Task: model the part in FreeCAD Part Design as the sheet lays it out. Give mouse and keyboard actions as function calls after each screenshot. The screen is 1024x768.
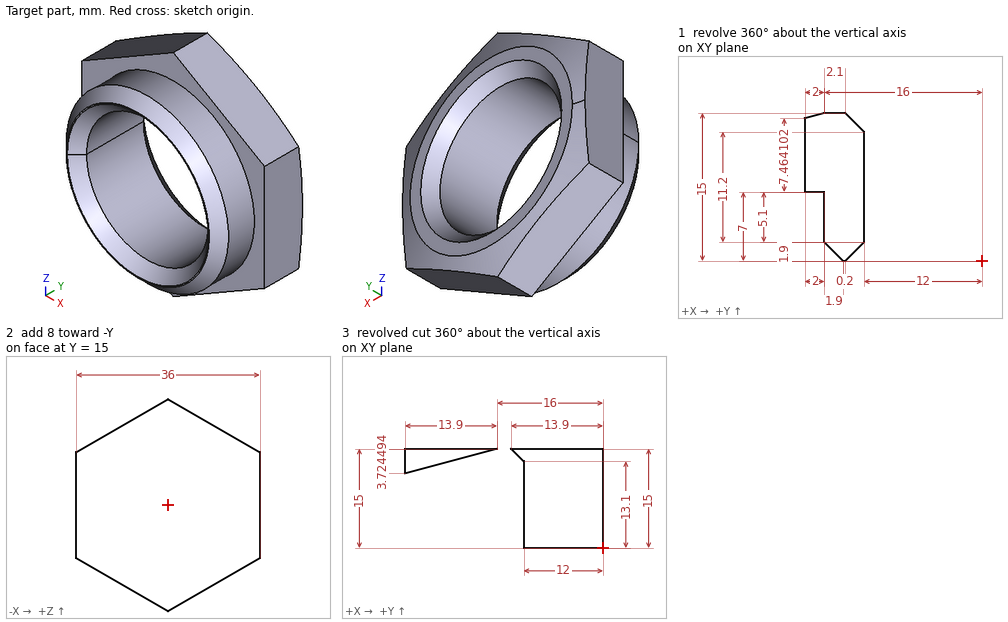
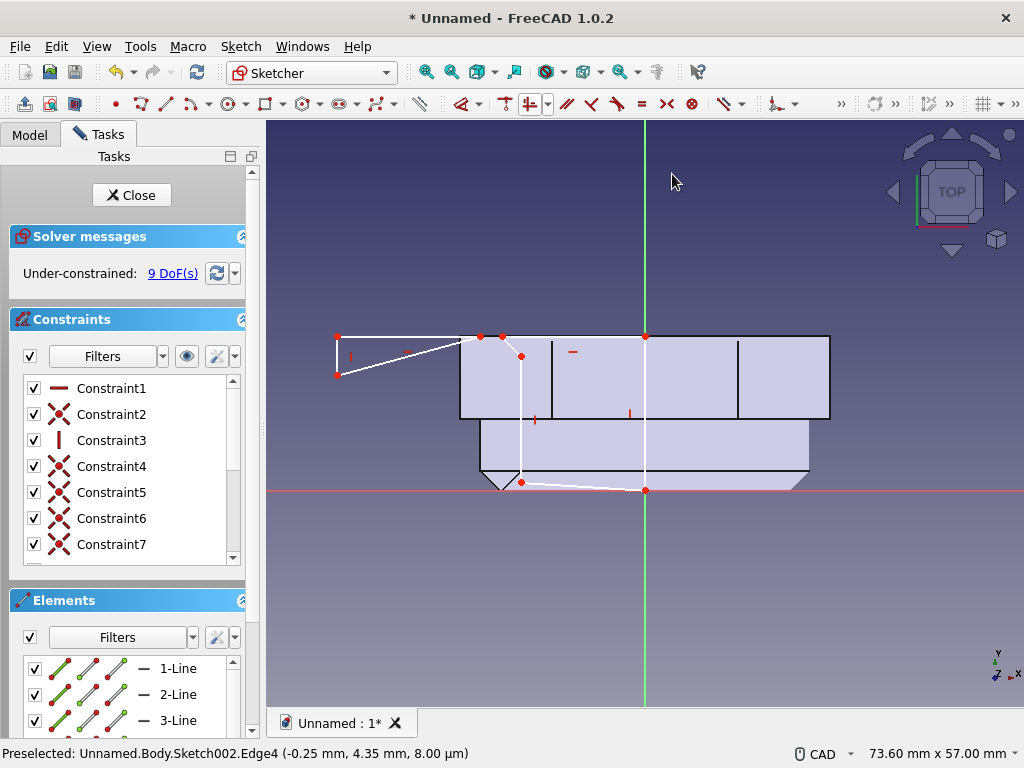
click(608, 488)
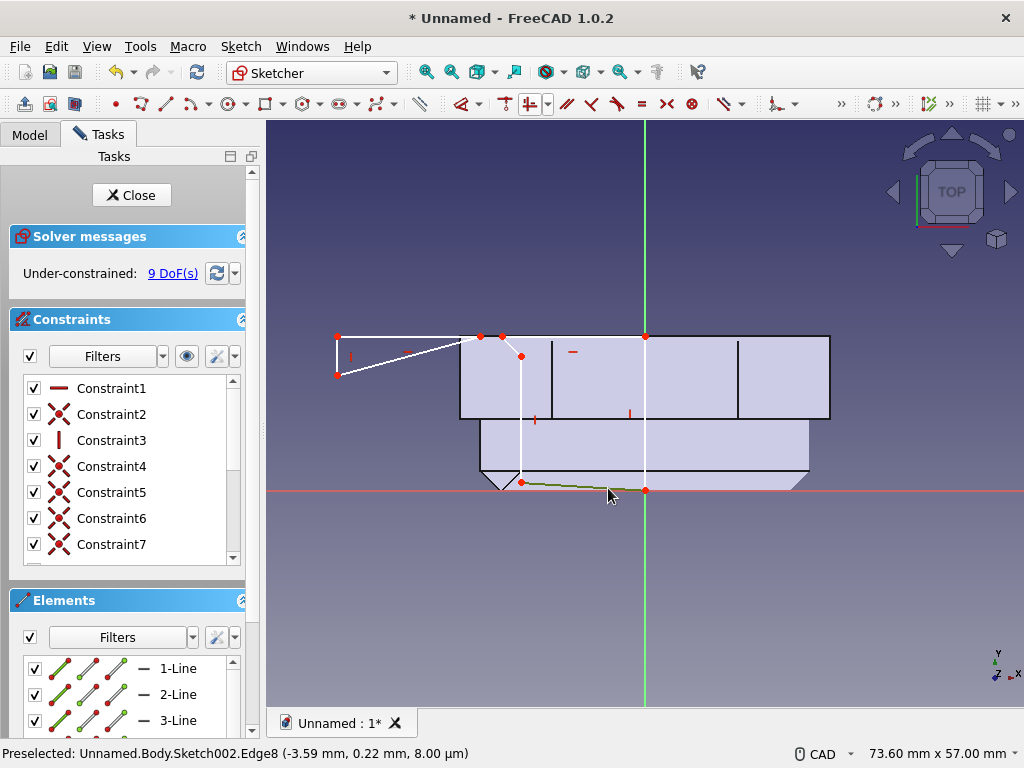
key(h)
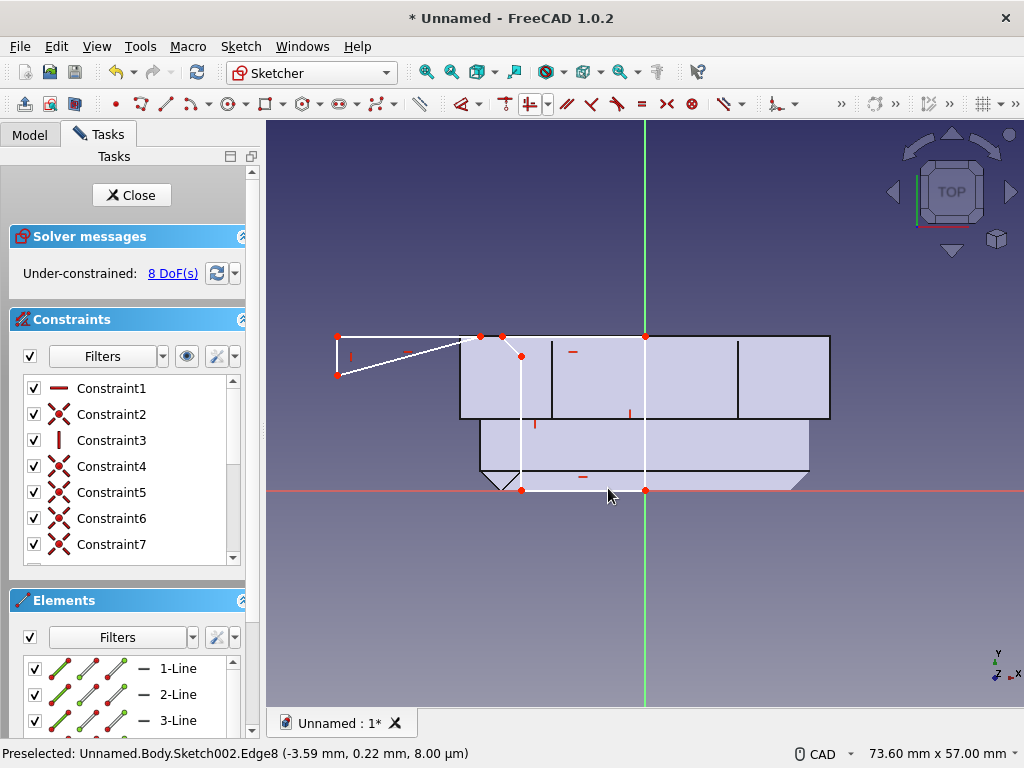
click(460, 104)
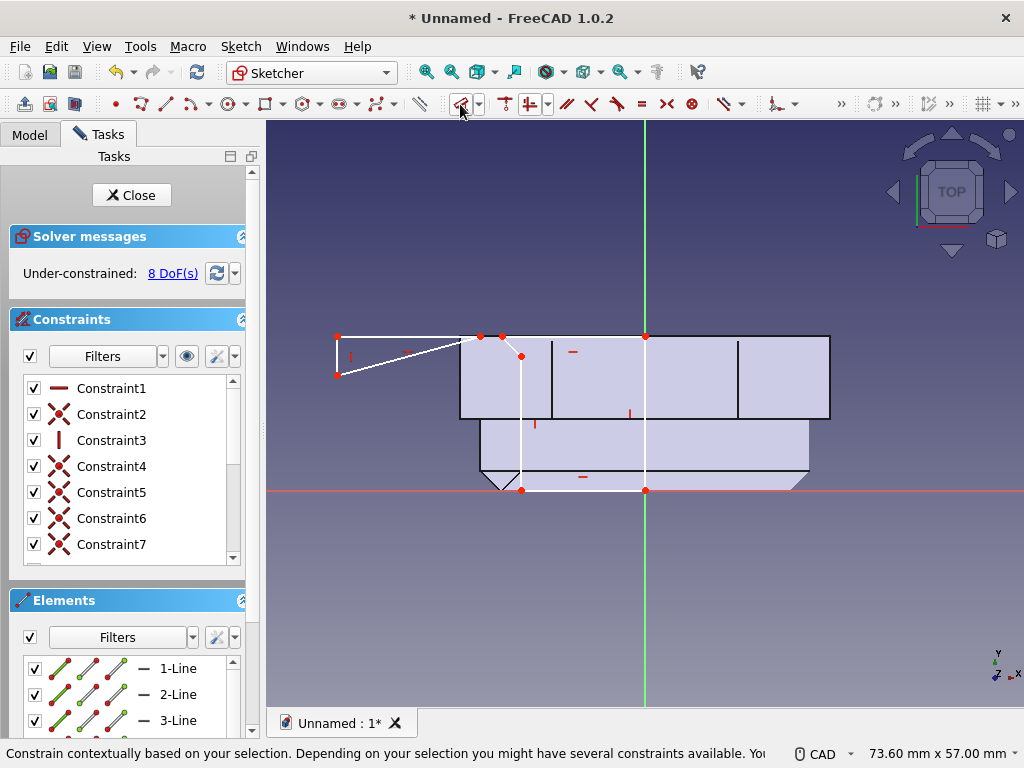
click(645, 445)
click(679, 414)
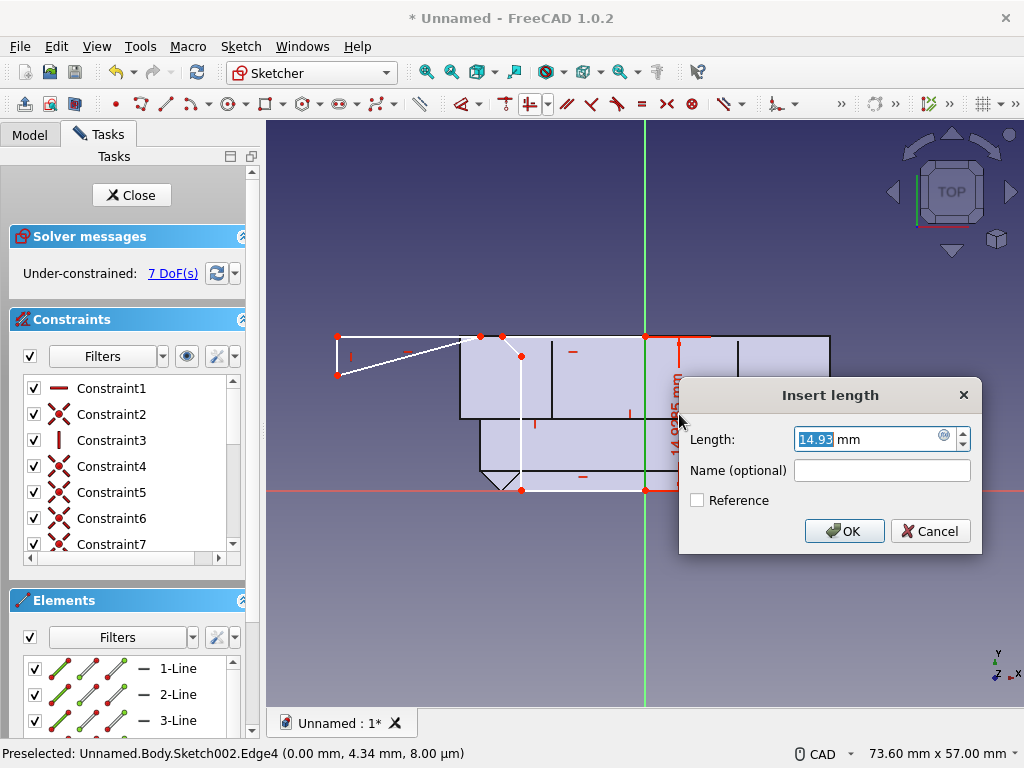
text(15)
key(Return)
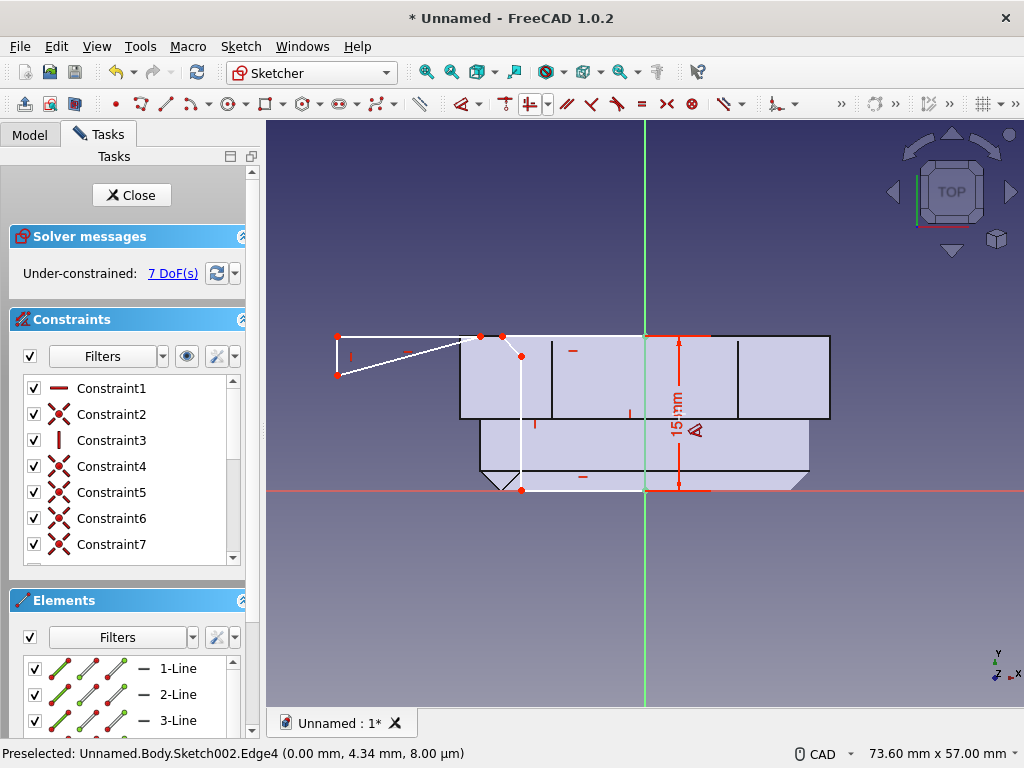
click(558, 491)
click(583, 525)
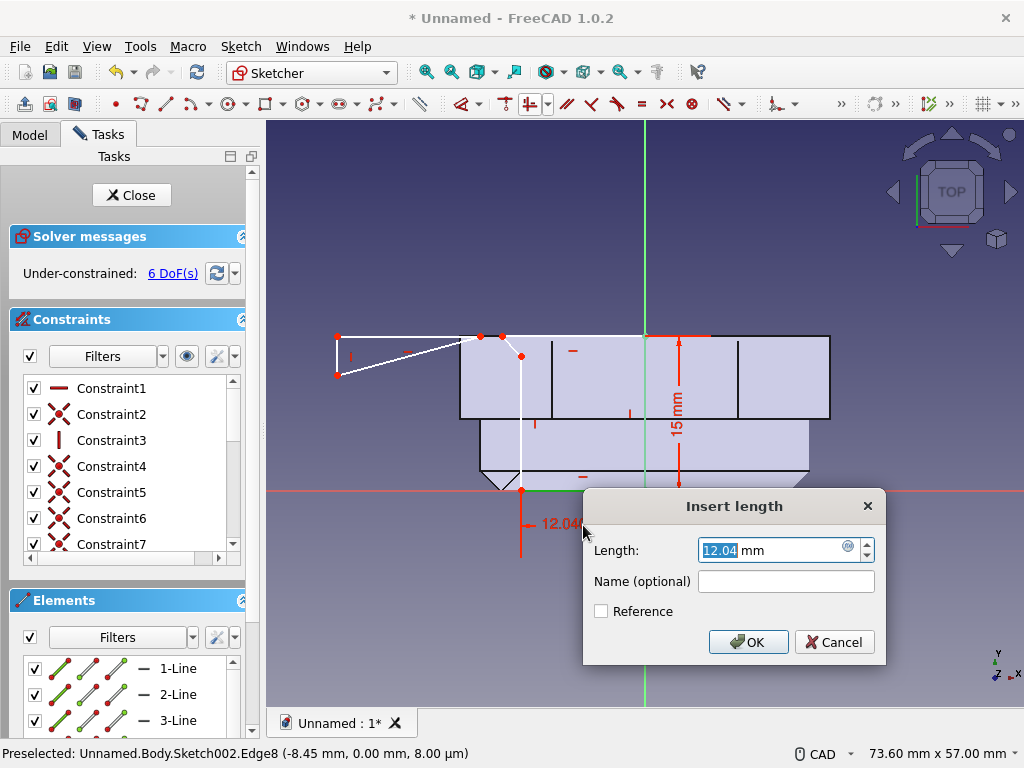
text(12)
key(Return)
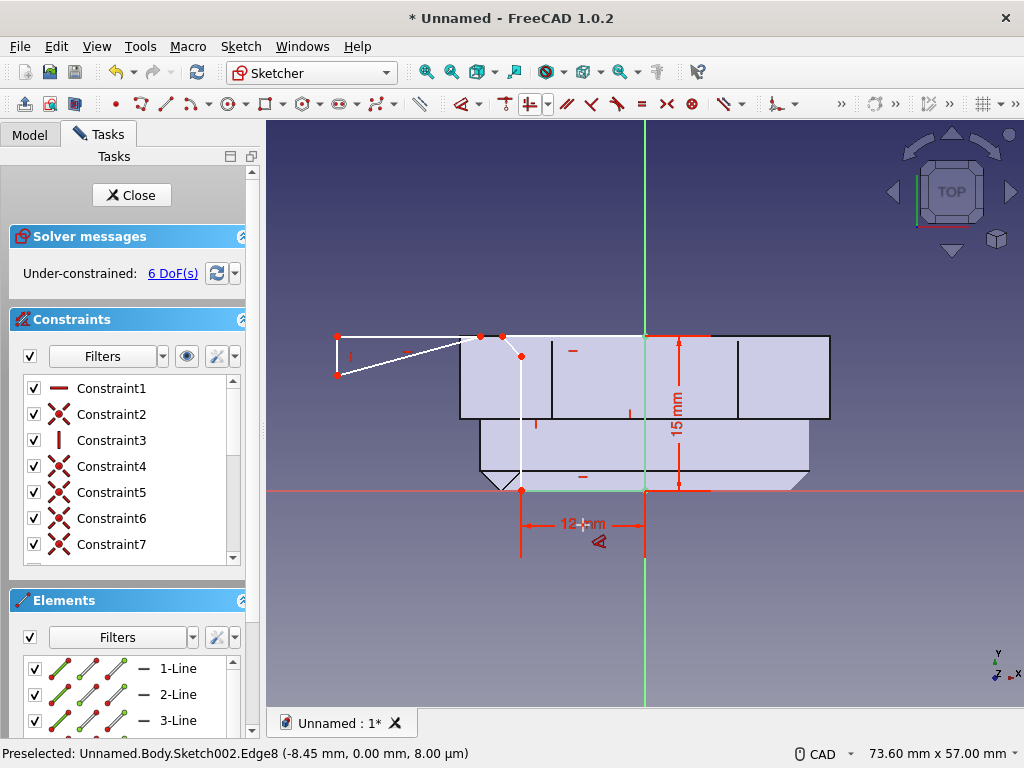
click(480, 337)
click(505, 525)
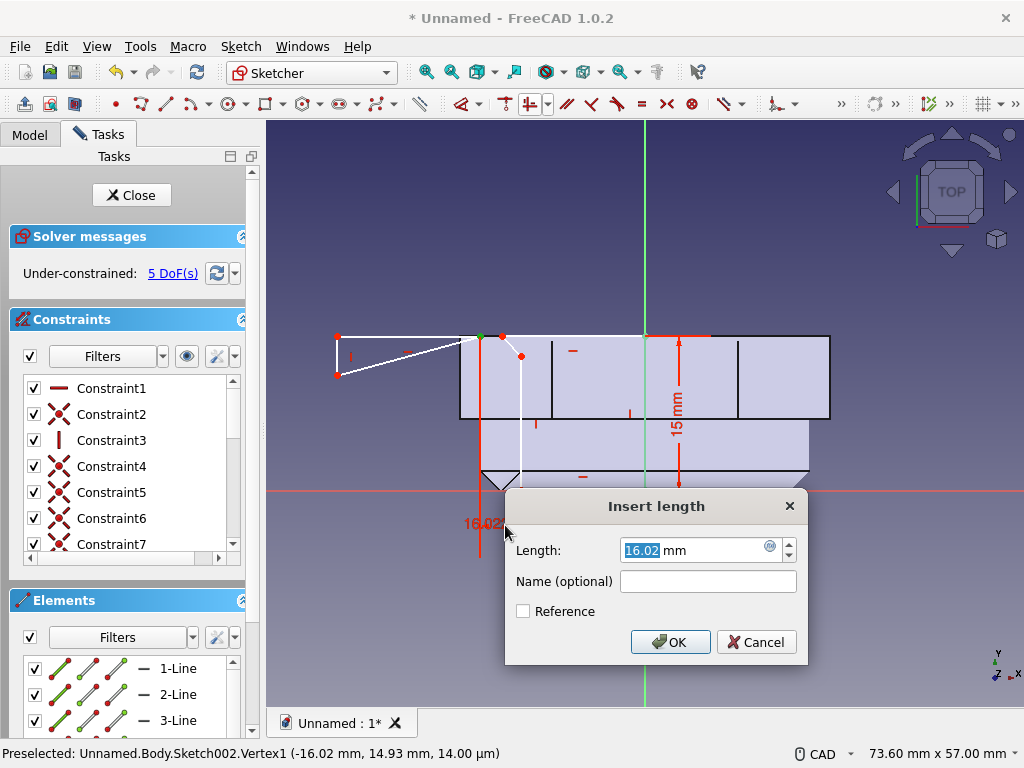
text(16)
key(Return)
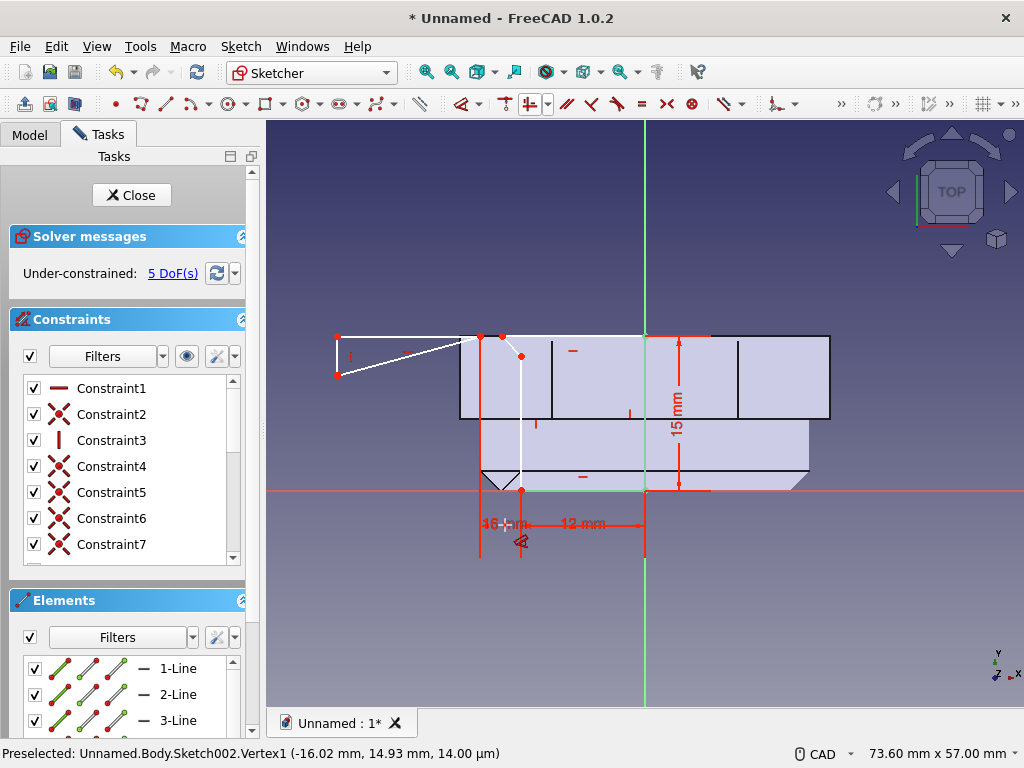
click(480, 337)
click(679, 379)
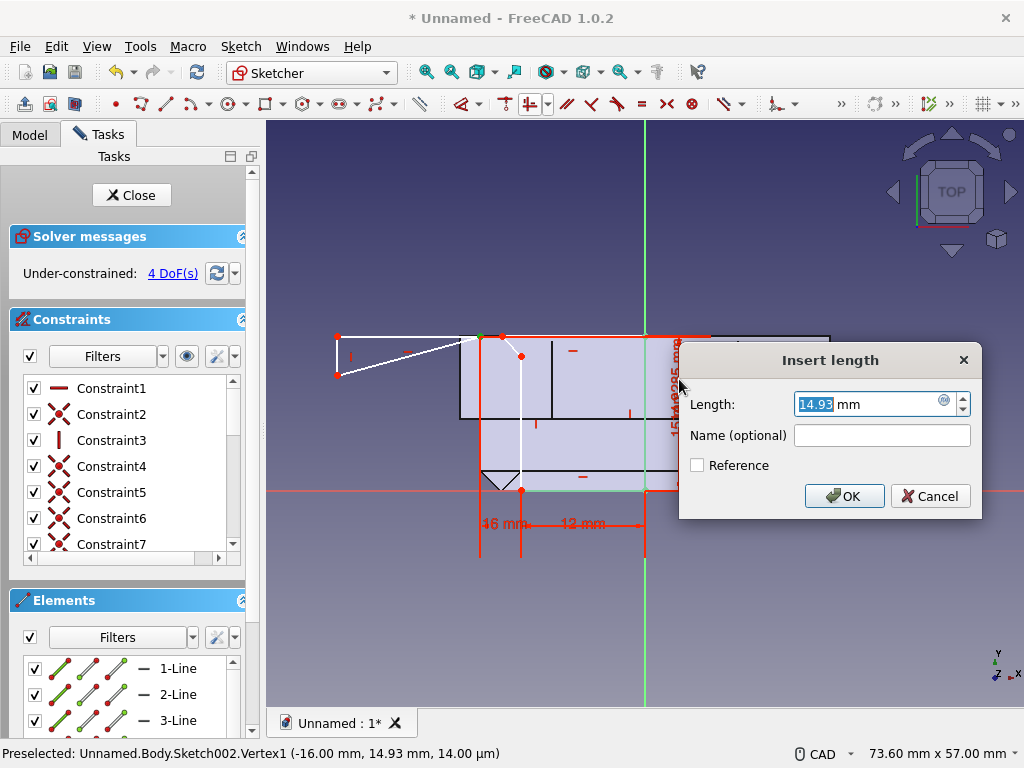
text(15)
key(Return)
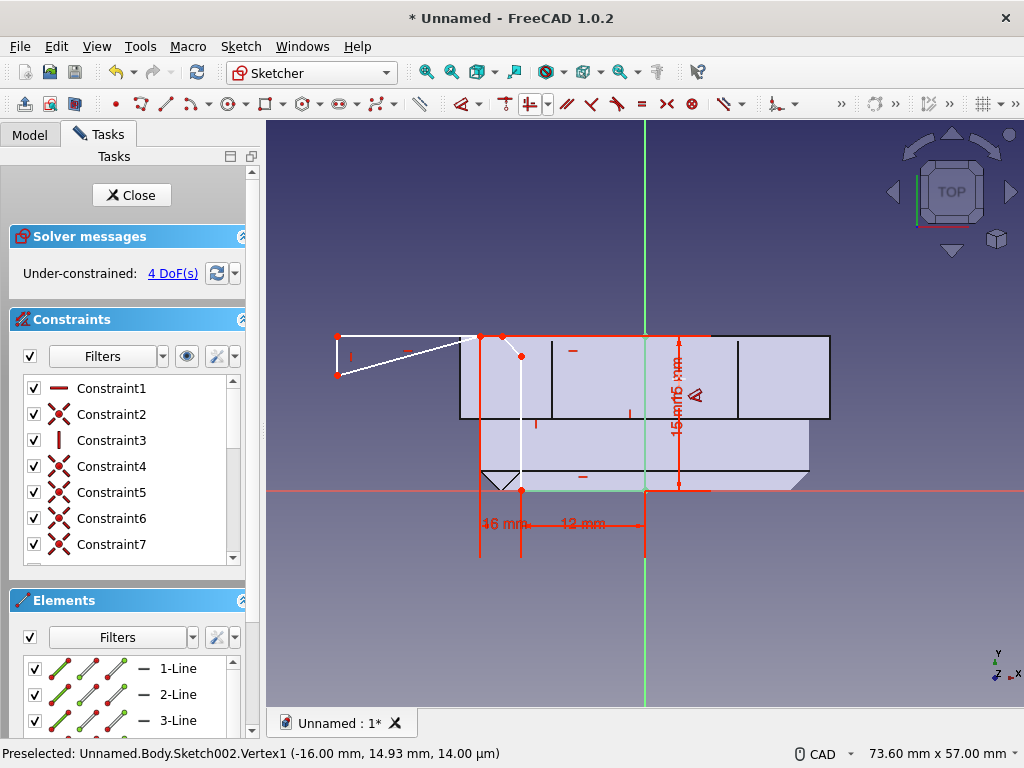
click(437, 336)
click(409, 302)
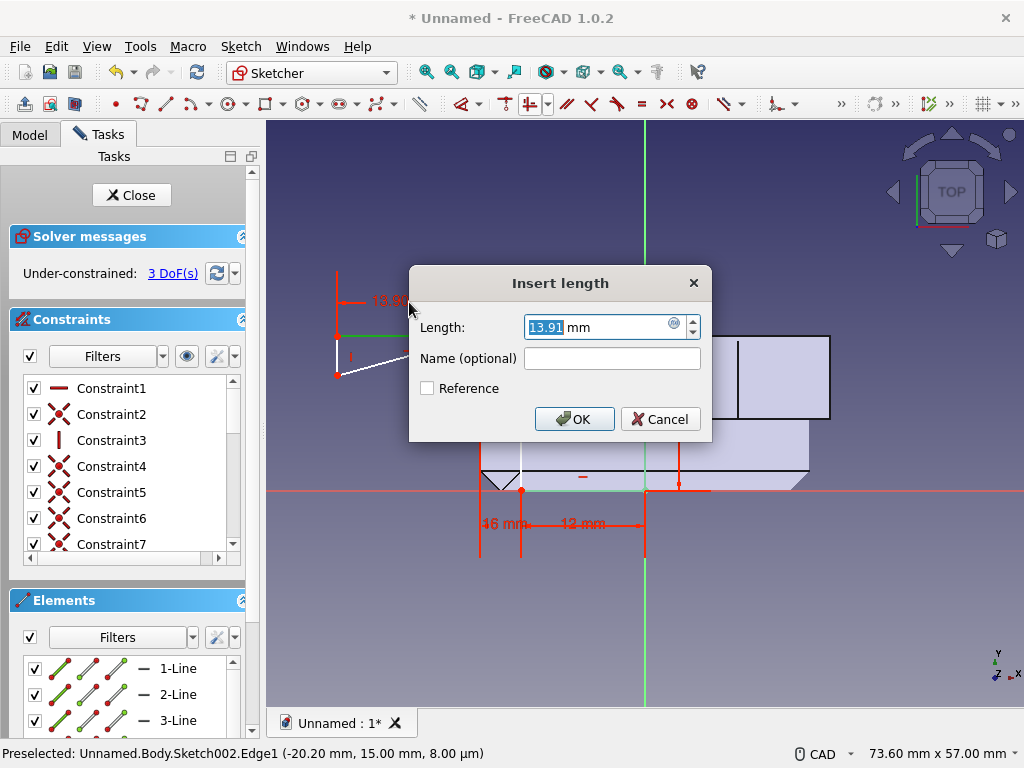
text(13.9)
key(Return)